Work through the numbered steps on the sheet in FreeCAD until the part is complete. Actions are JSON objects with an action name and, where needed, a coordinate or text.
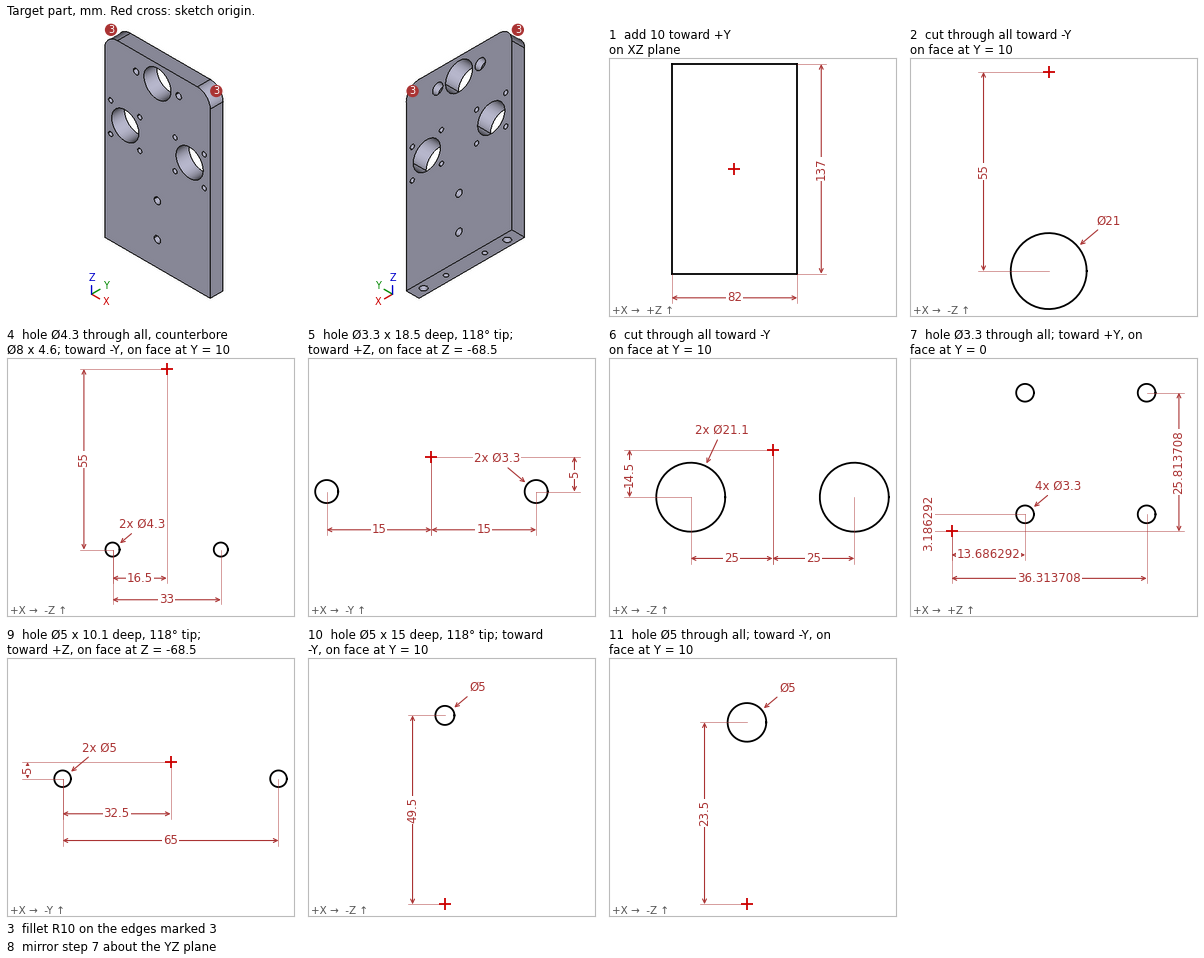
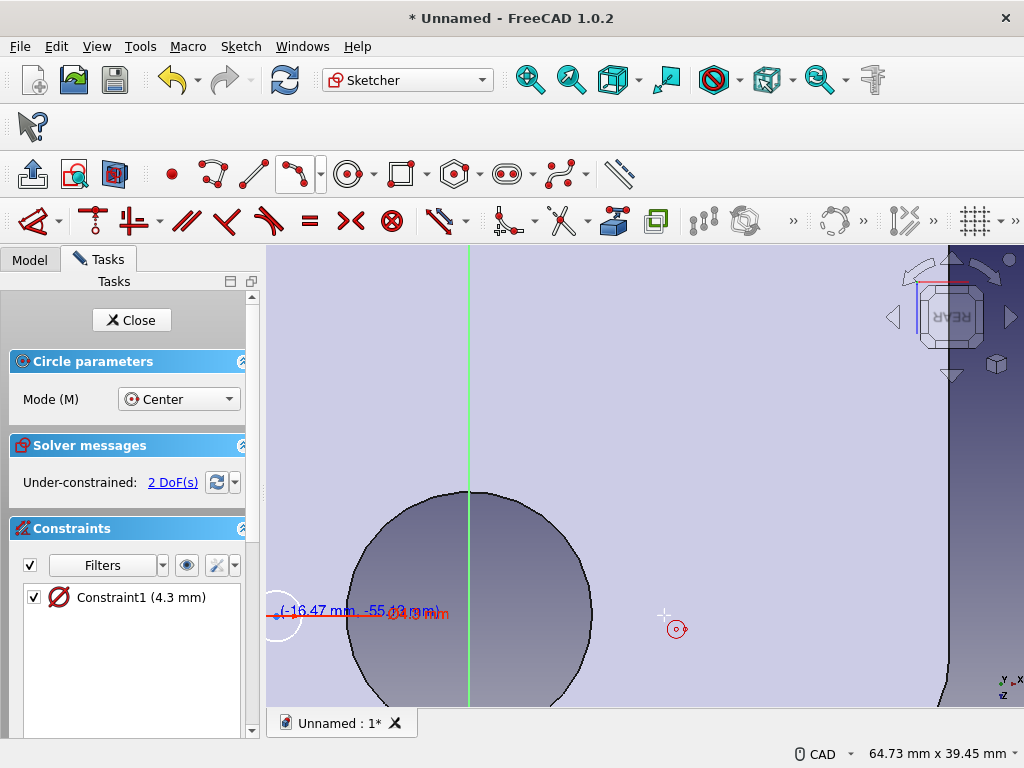
{"action": "left_click", "coordinate": [663, 615]}
{"action": "mouse_move", "coordinate": [680, 597]}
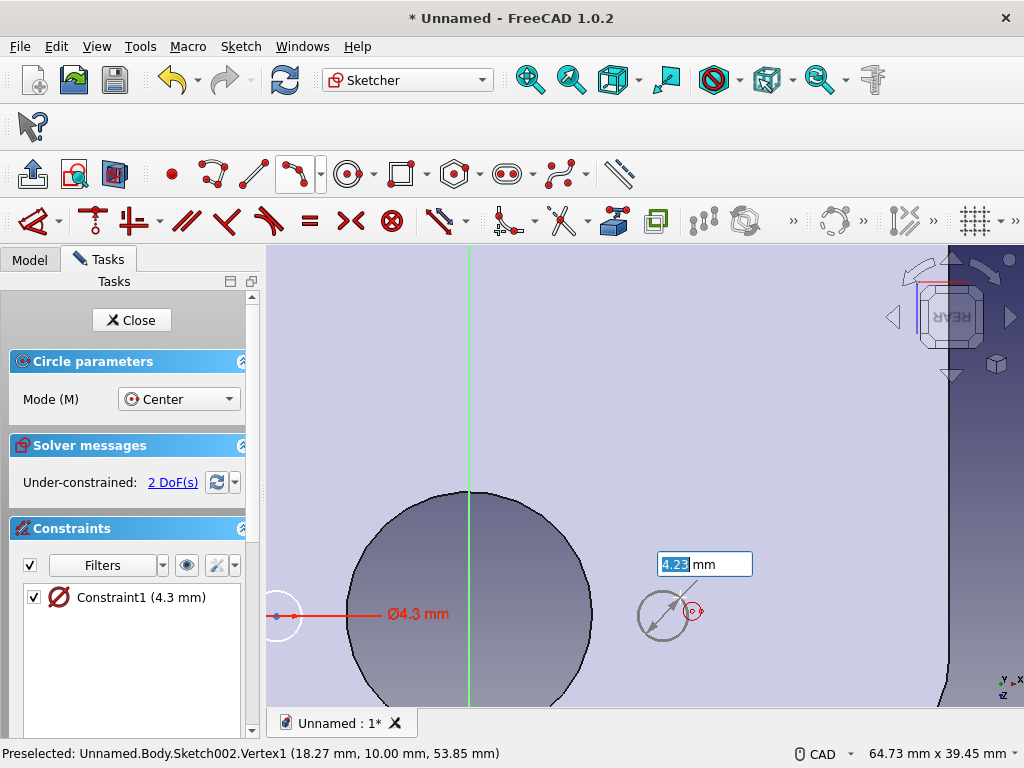
{"action": "type", "text": "4.3"}
{"action": "key", "text": "Return"}
{"action": "key", "text": "Escape"}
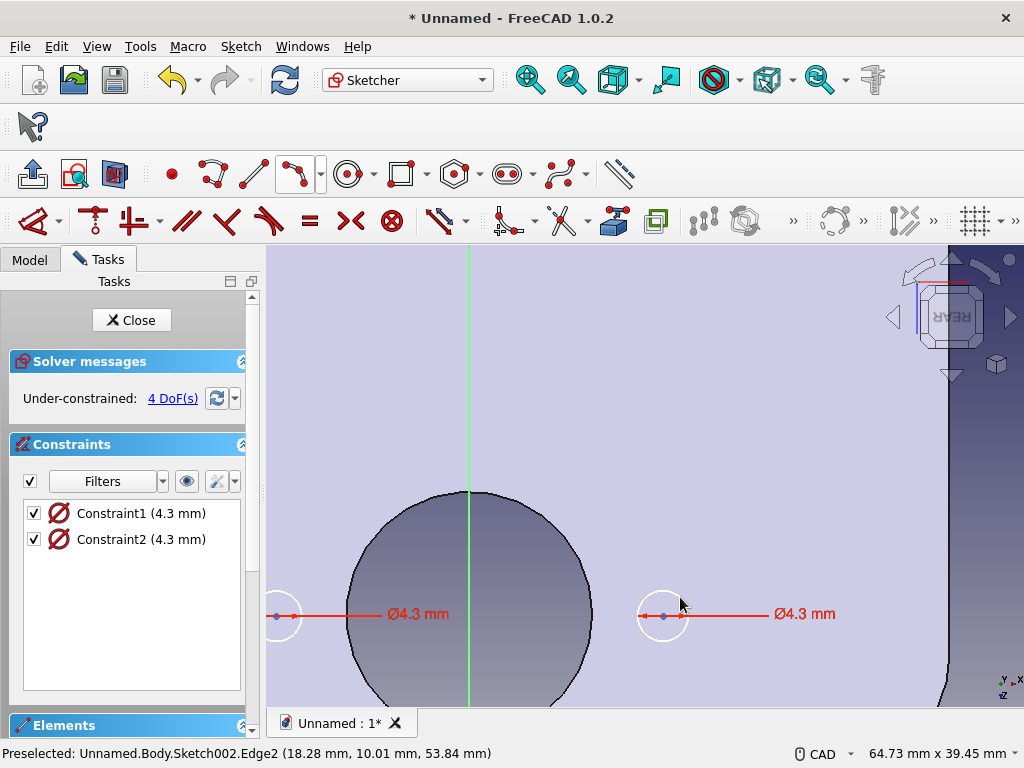
{"action": "scroll", "coordinate": [664, 615], "scroll_direction": "down", "scroll_amount": 4}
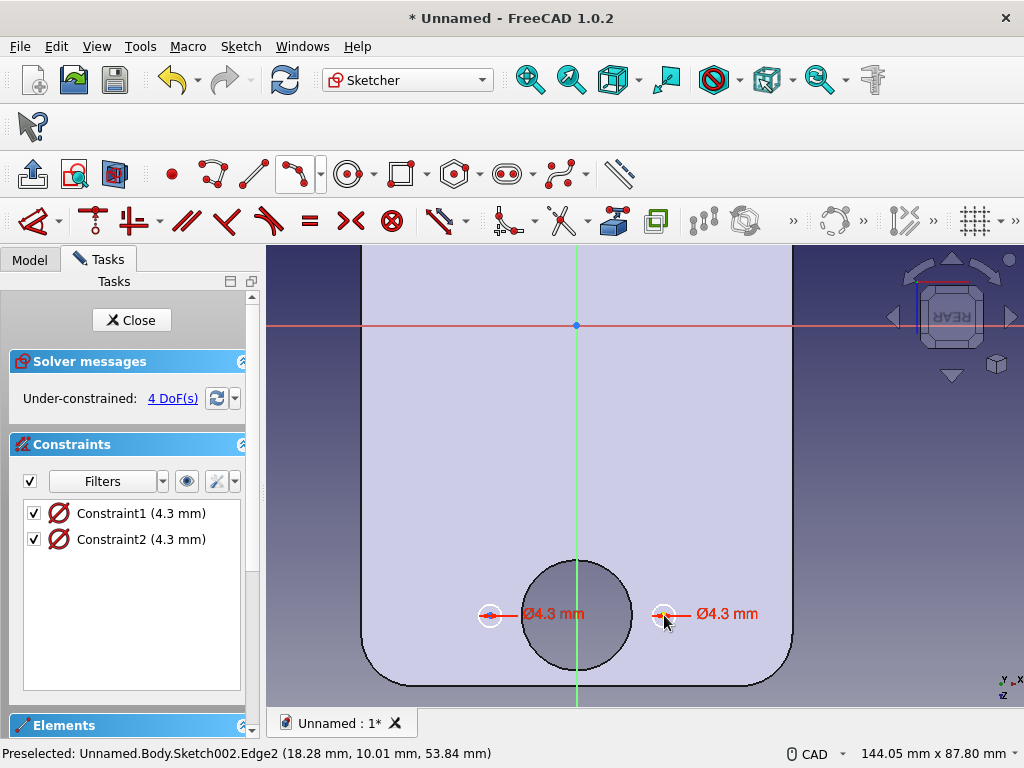
{"action": "left_click", "coordinate": [490, 616]}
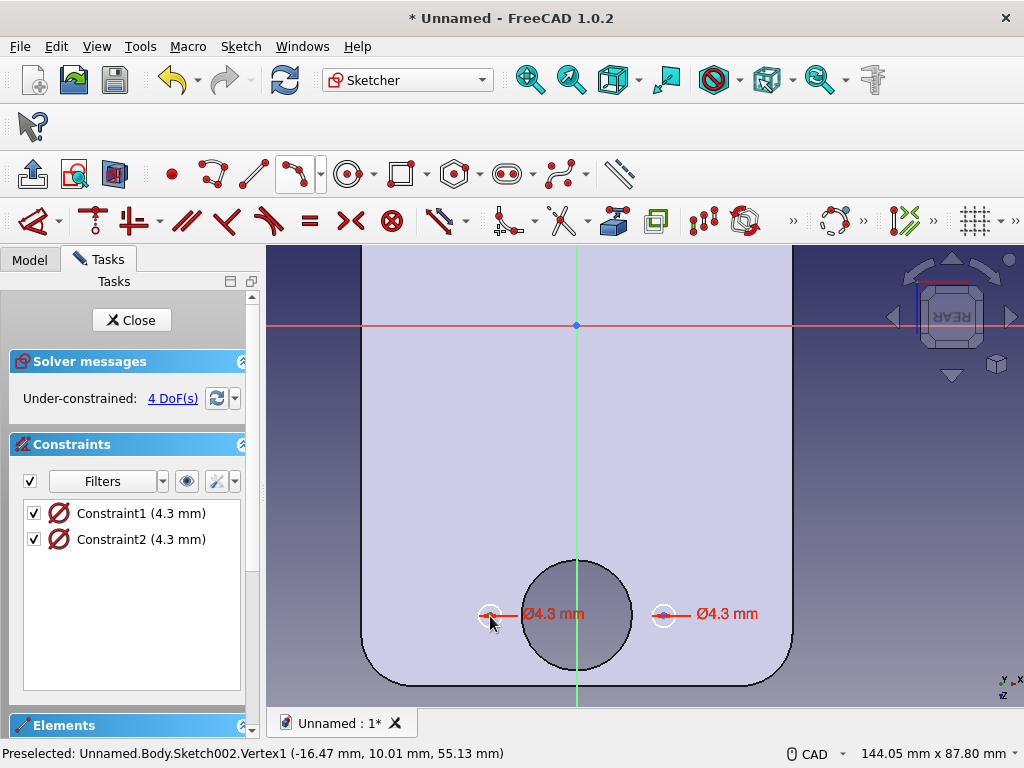
{"action": "left_click", "coordinate": [664, 616]}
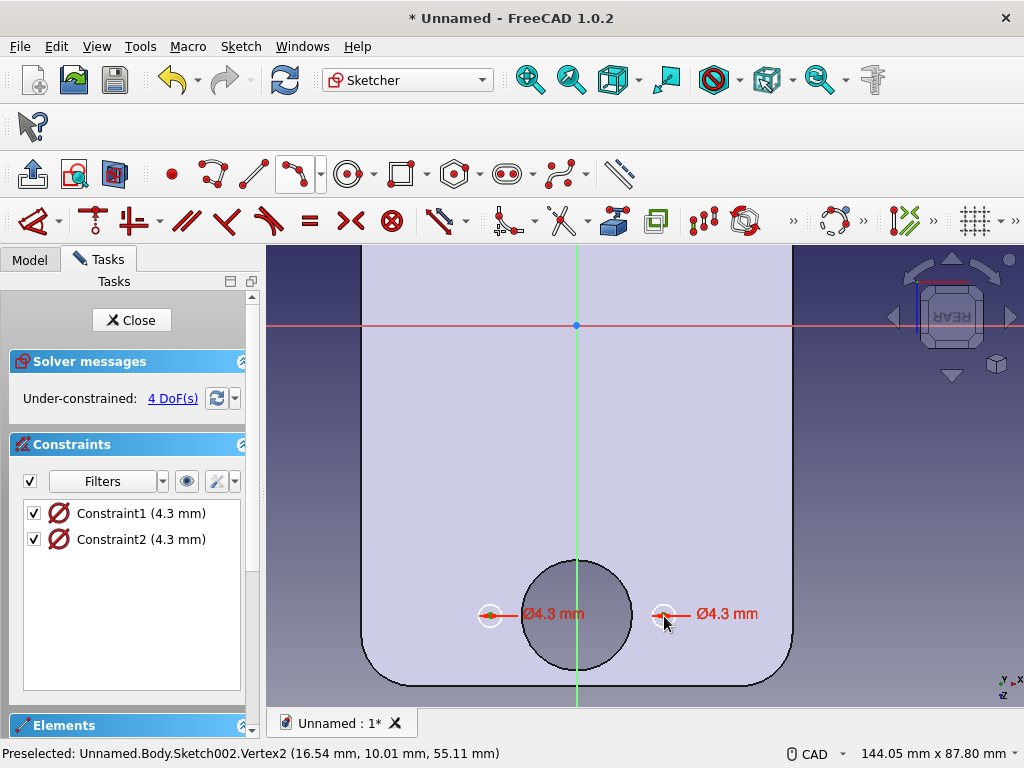
{"action": "key", "text": "h"}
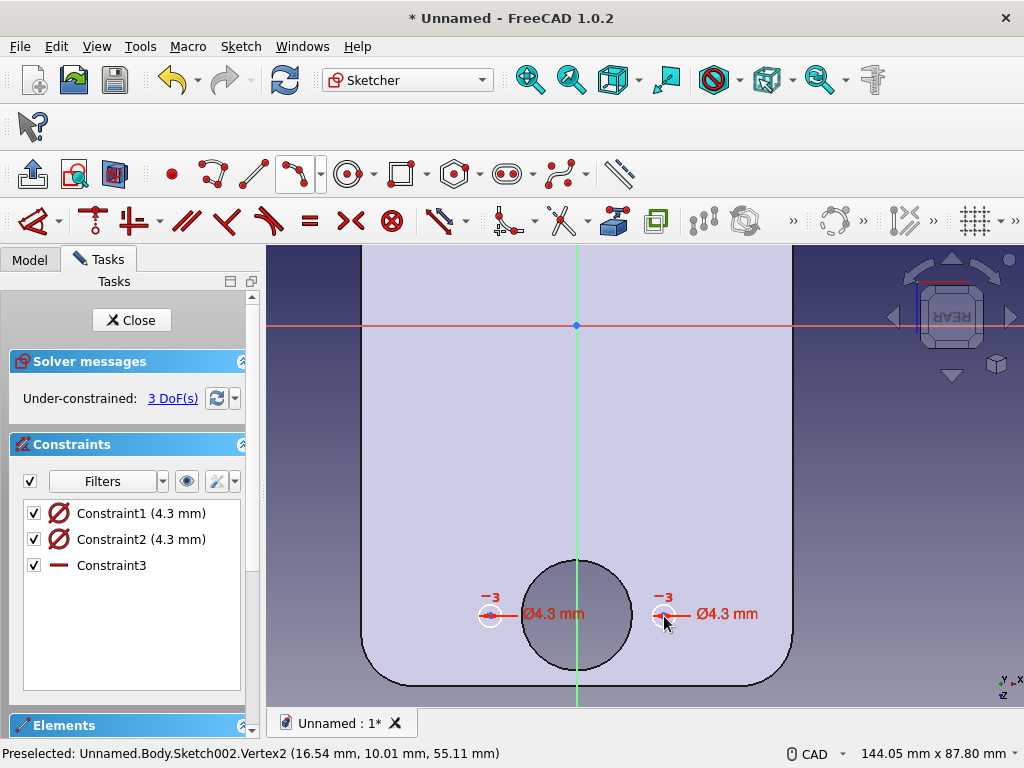
{"action": "left_click", "coordinate": [32, 222]}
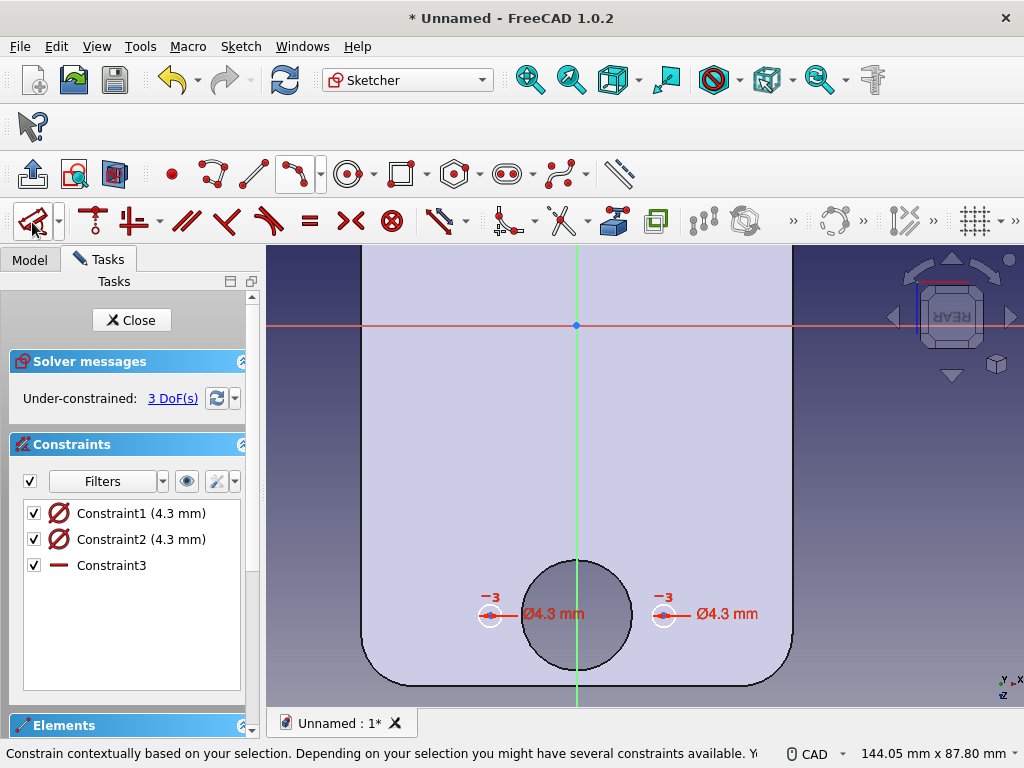
{"action": "left_click", "coordinate": [490, 616]}
{"action": "left_click", "coordinate": [456, 471]}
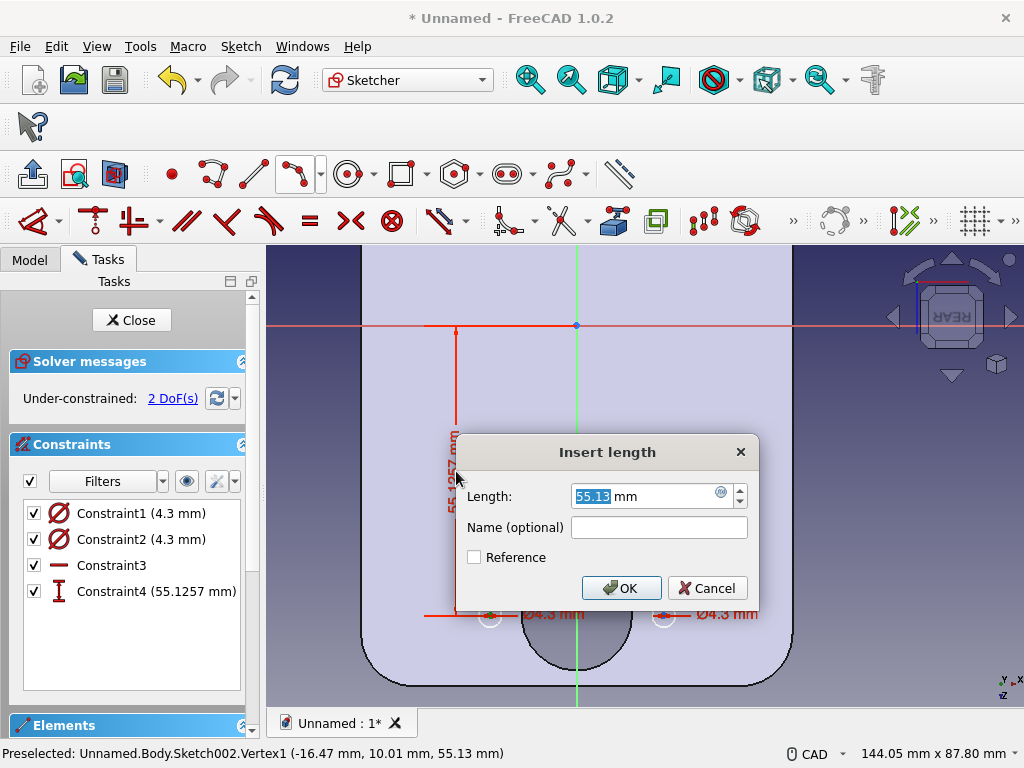
{"action": "type", "text": "55"}
{"action": "key", "text": "Return"}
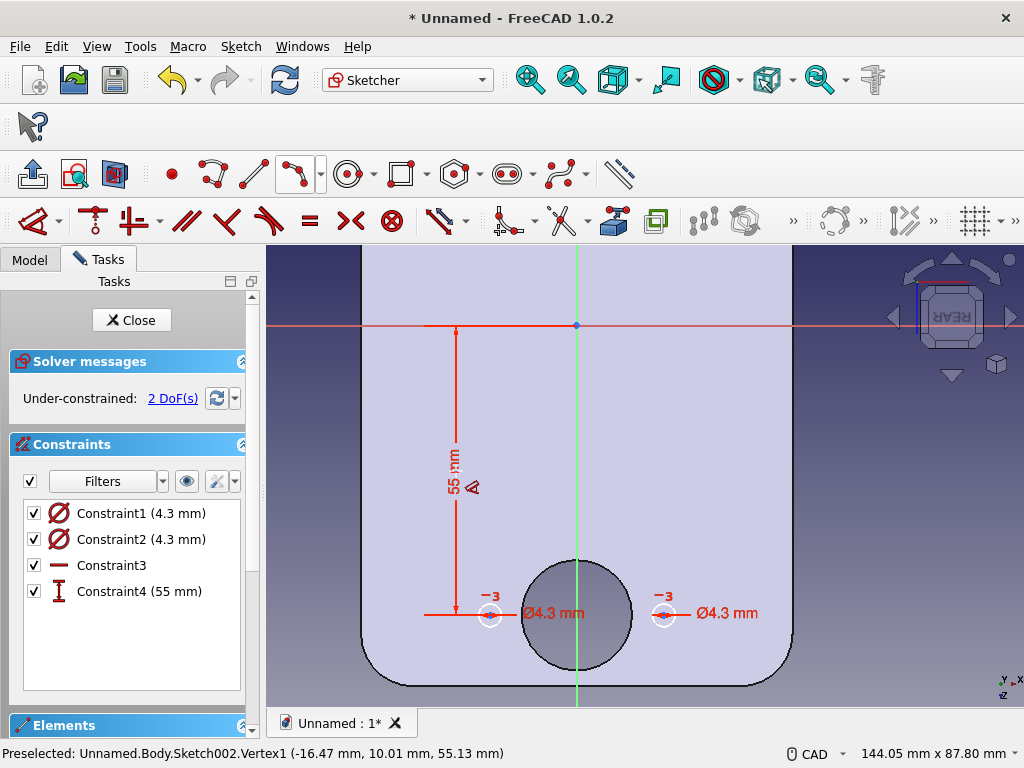
{"action": "left_click", "coordinate": [490, 615]}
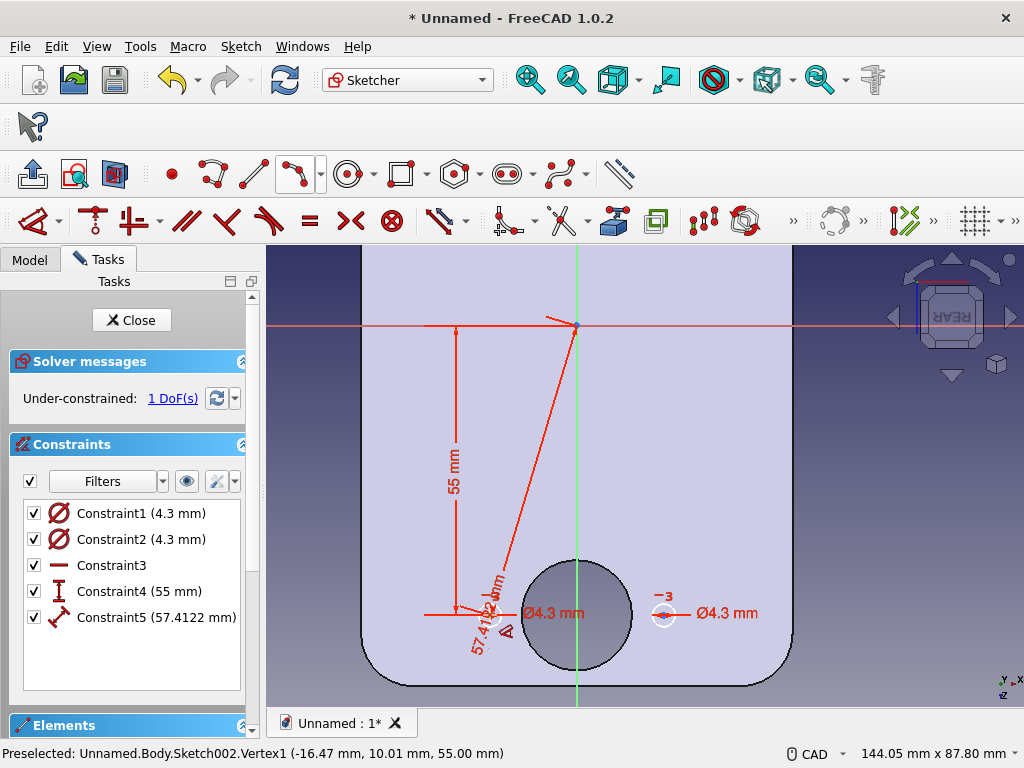
{"action": "left_click", "coordinate": [664, 615]}
{"action": "left_click", "coordinate": [537, 649]}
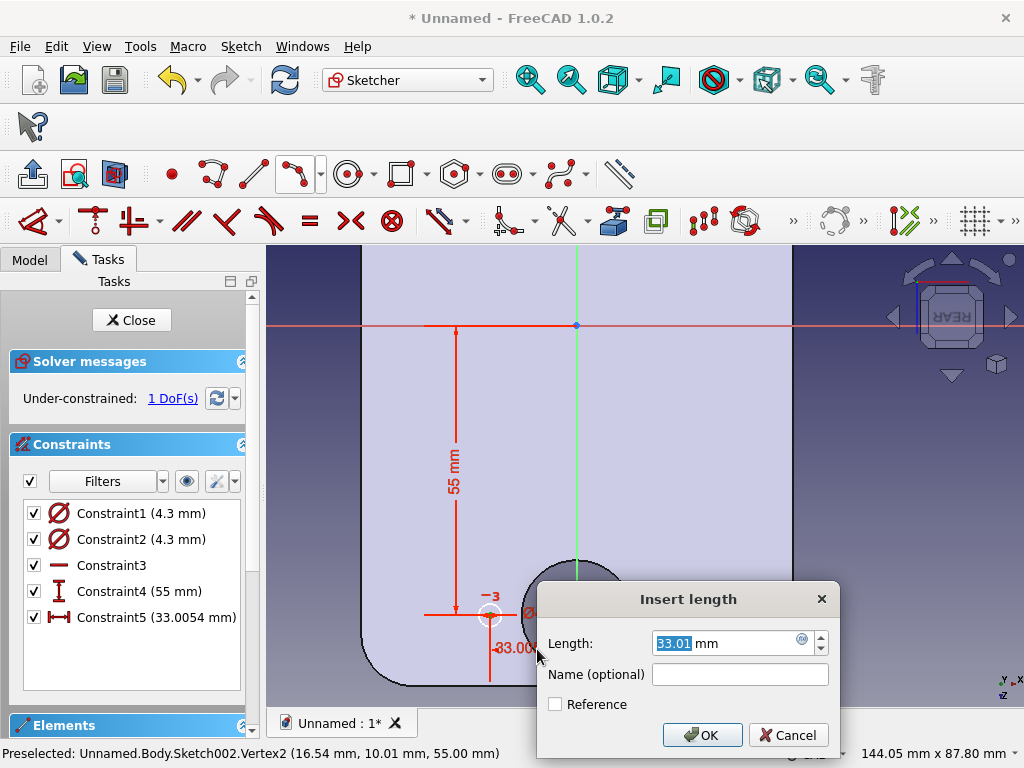
{"action": "type", "text": "33"}
{"action": "key", "text": "Return"}